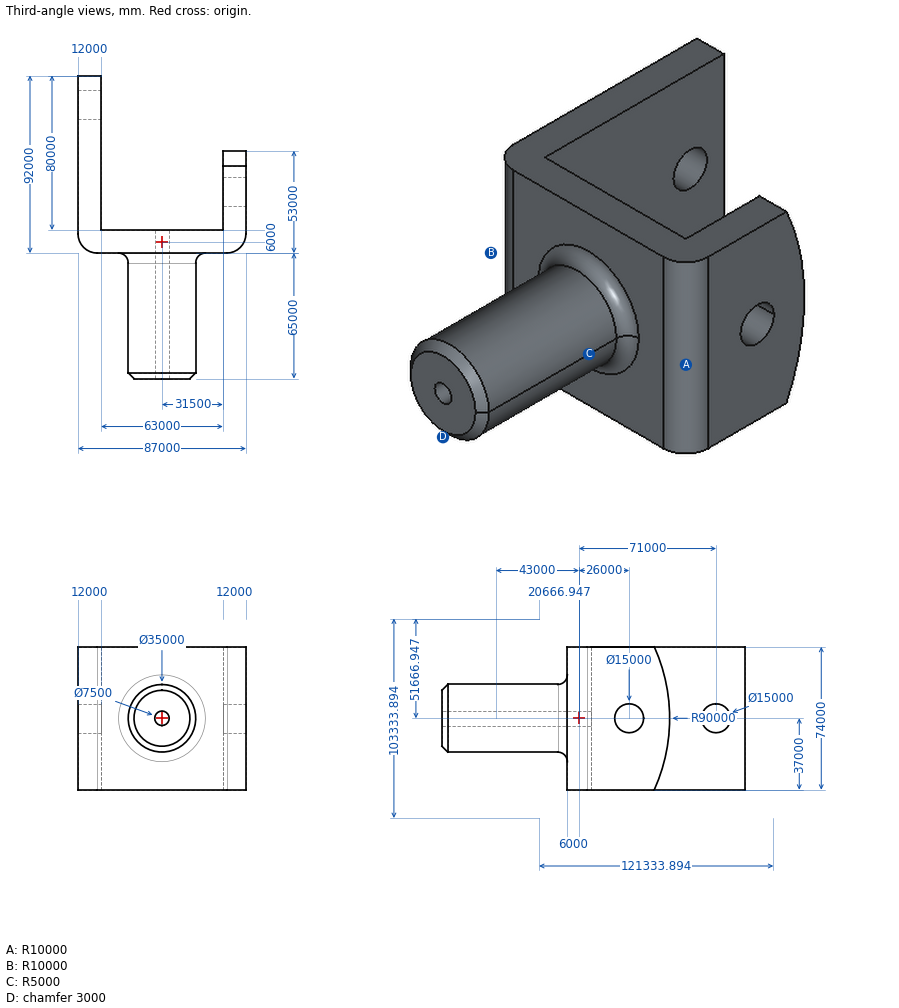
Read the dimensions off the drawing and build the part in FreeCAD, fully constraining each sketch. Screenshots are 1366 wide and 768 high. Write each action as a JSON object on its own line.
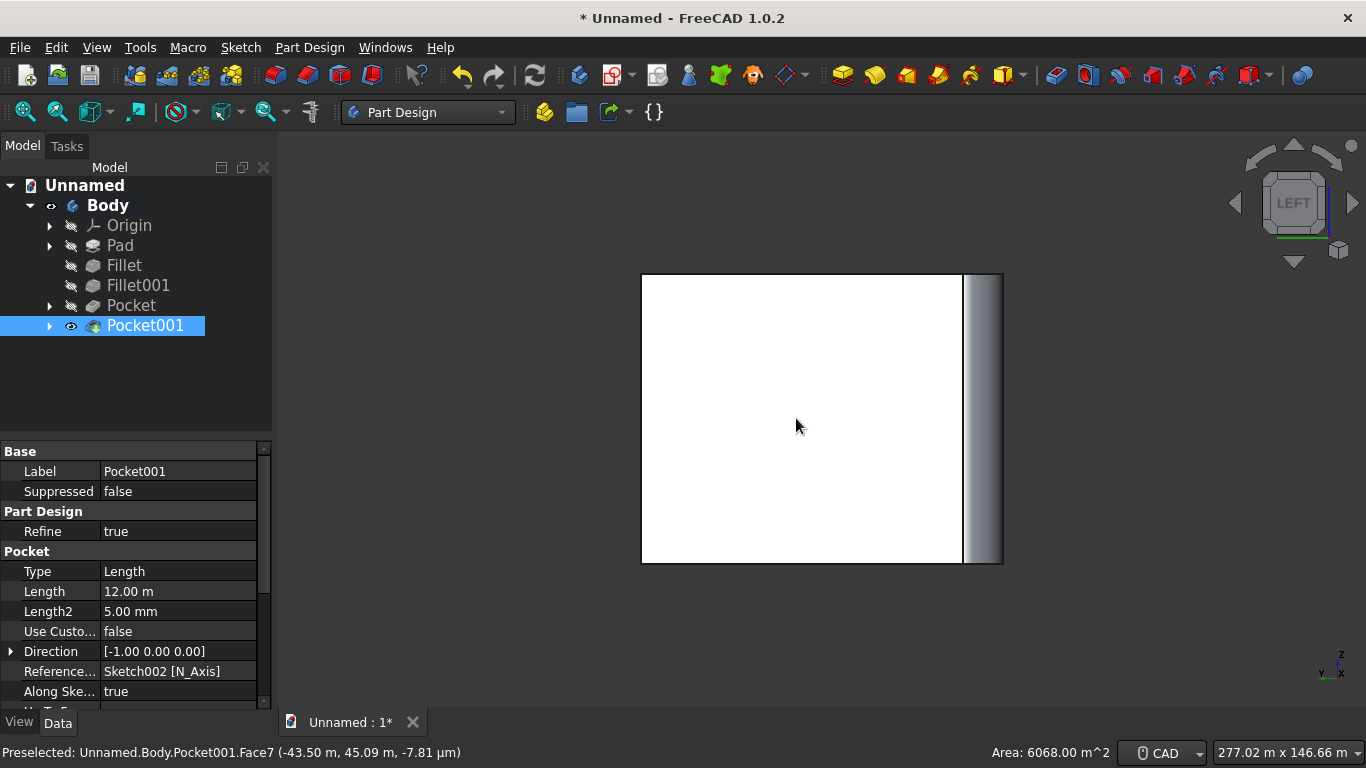
{"action": "left_click", "coordinate": [612, 76]}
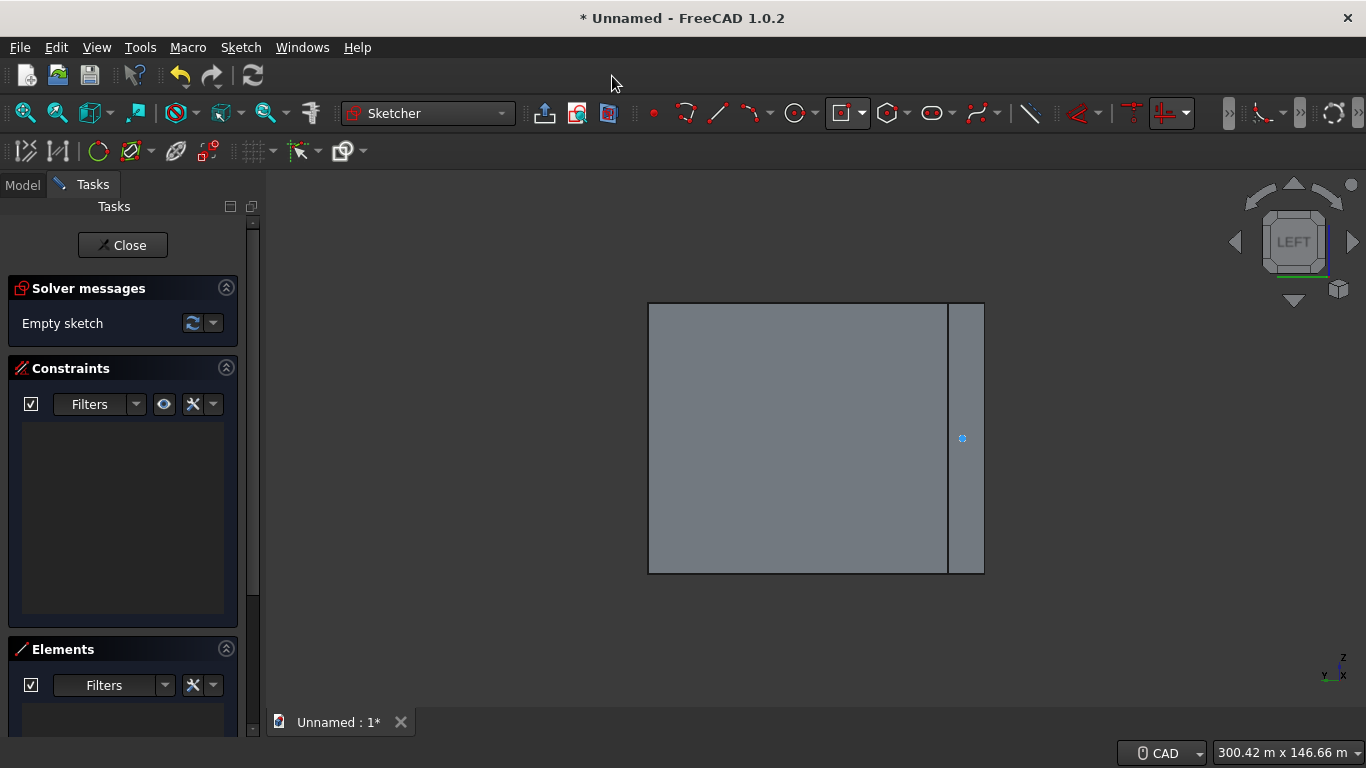
{"action": "scroll", "coordinate": [694, 438], "scroll_direction": "up", "scroll_amount": 9}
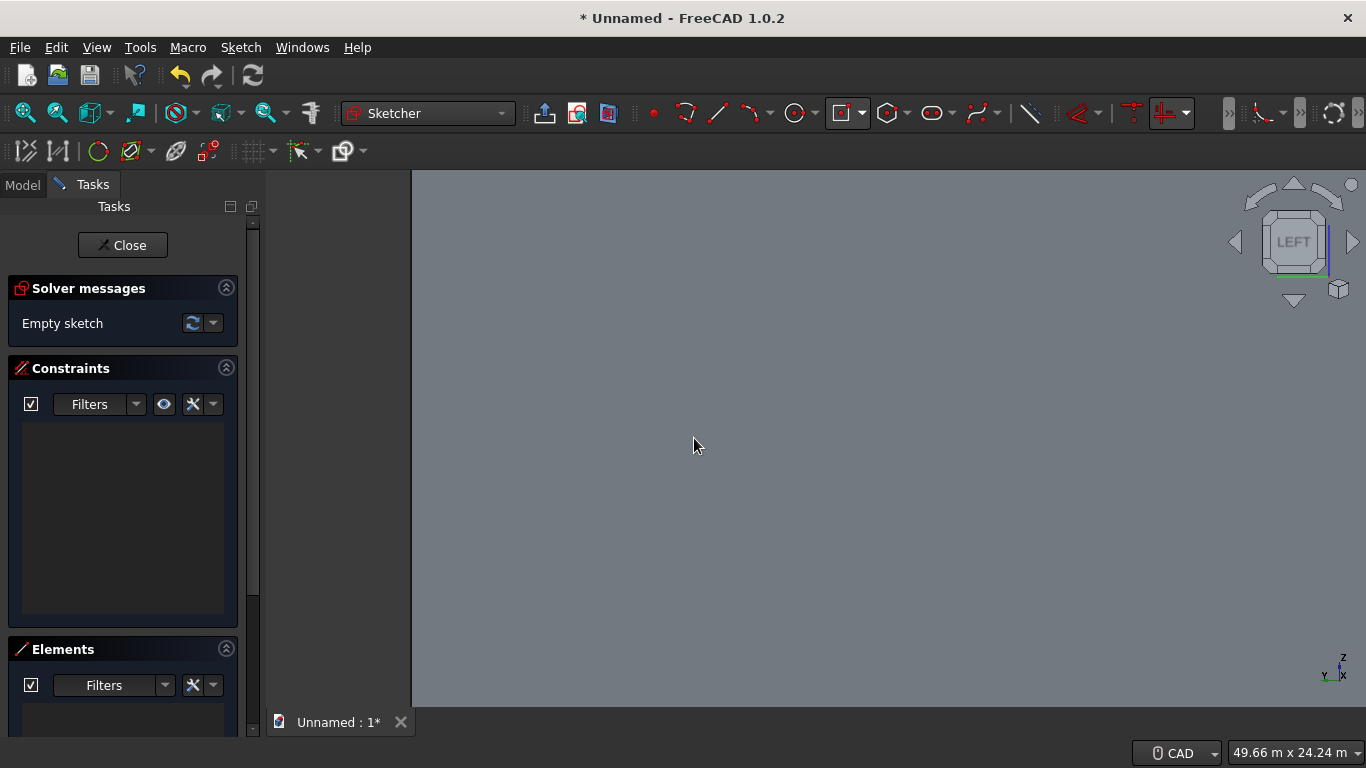
{"action": "key", "text": "g c"}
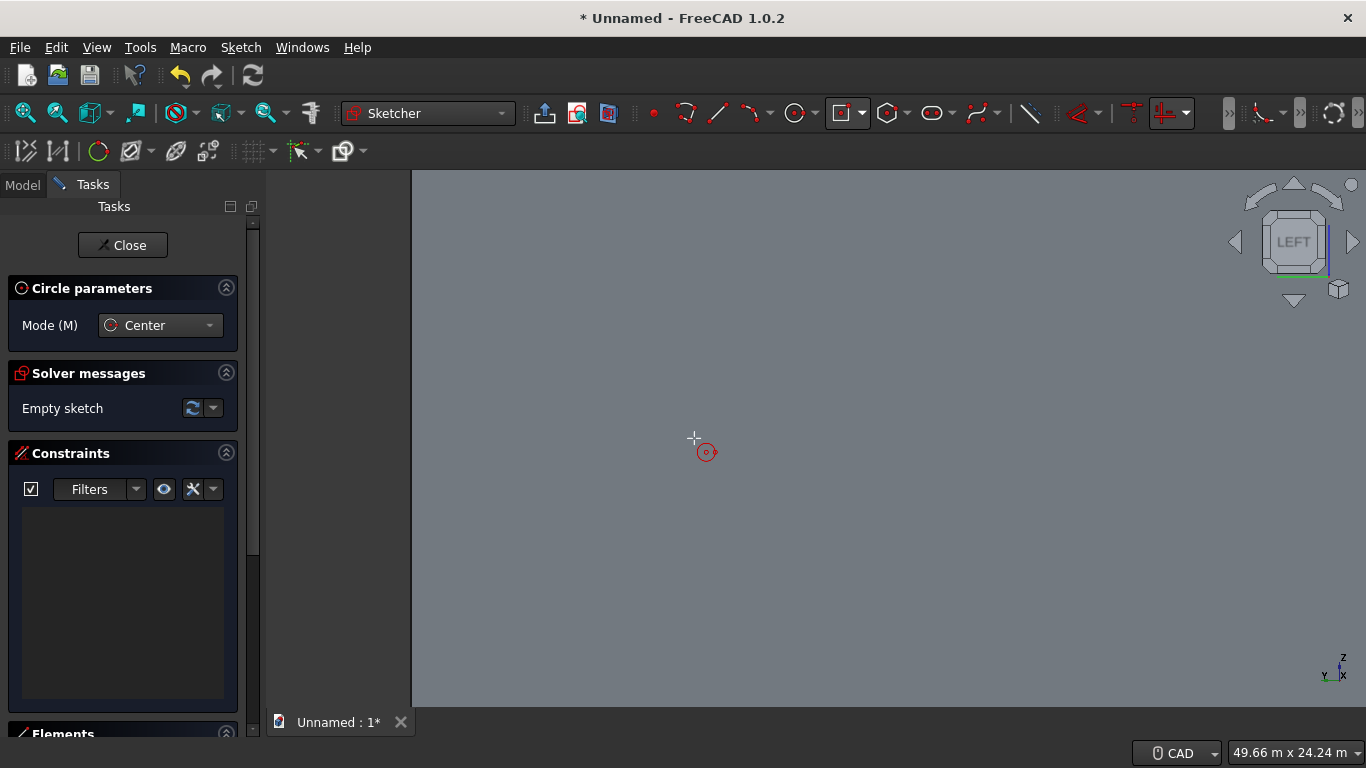
{"action": "left_click", "coordinate": [743, 438]}
{"action": "left_click", "coordinate": [861, 321]}
{"action": "key", "text": "Escape"}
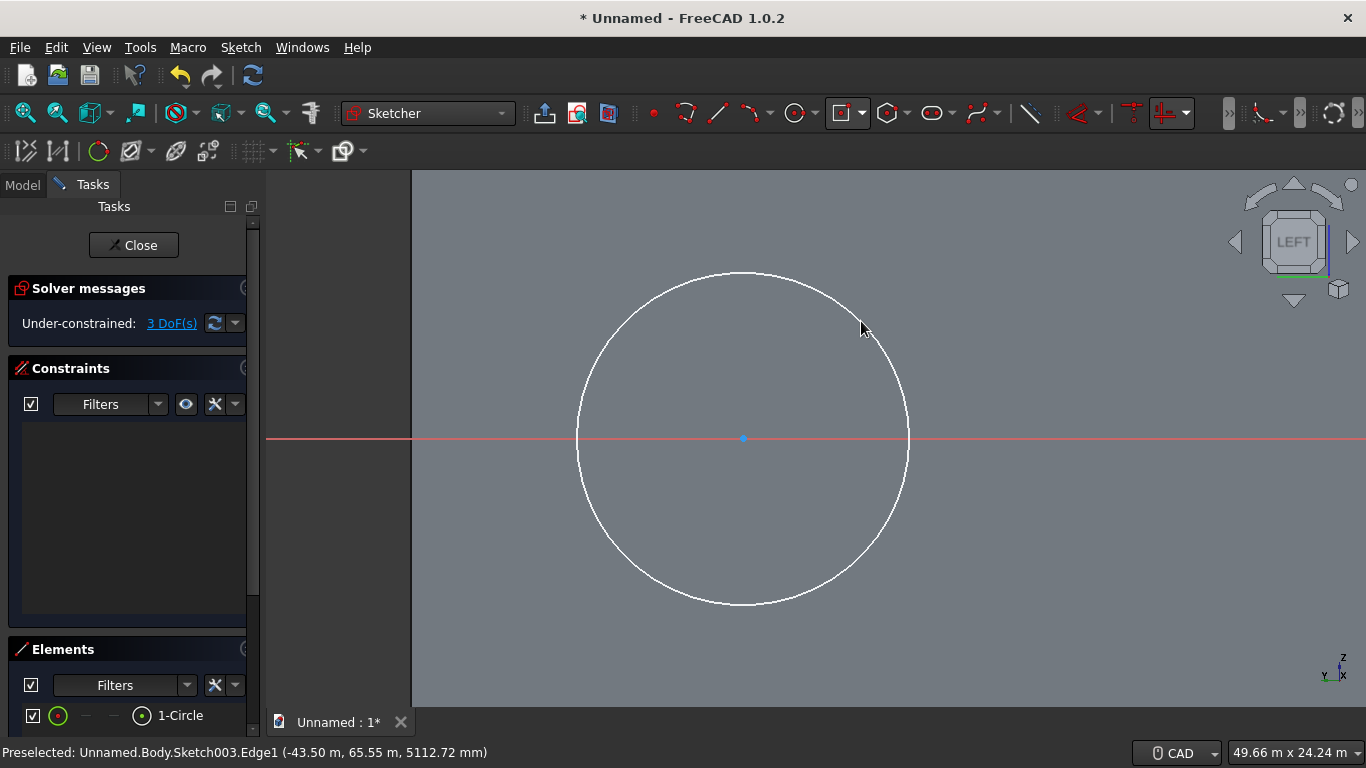
{"action": "left_click", "coordinate": [743, 439]}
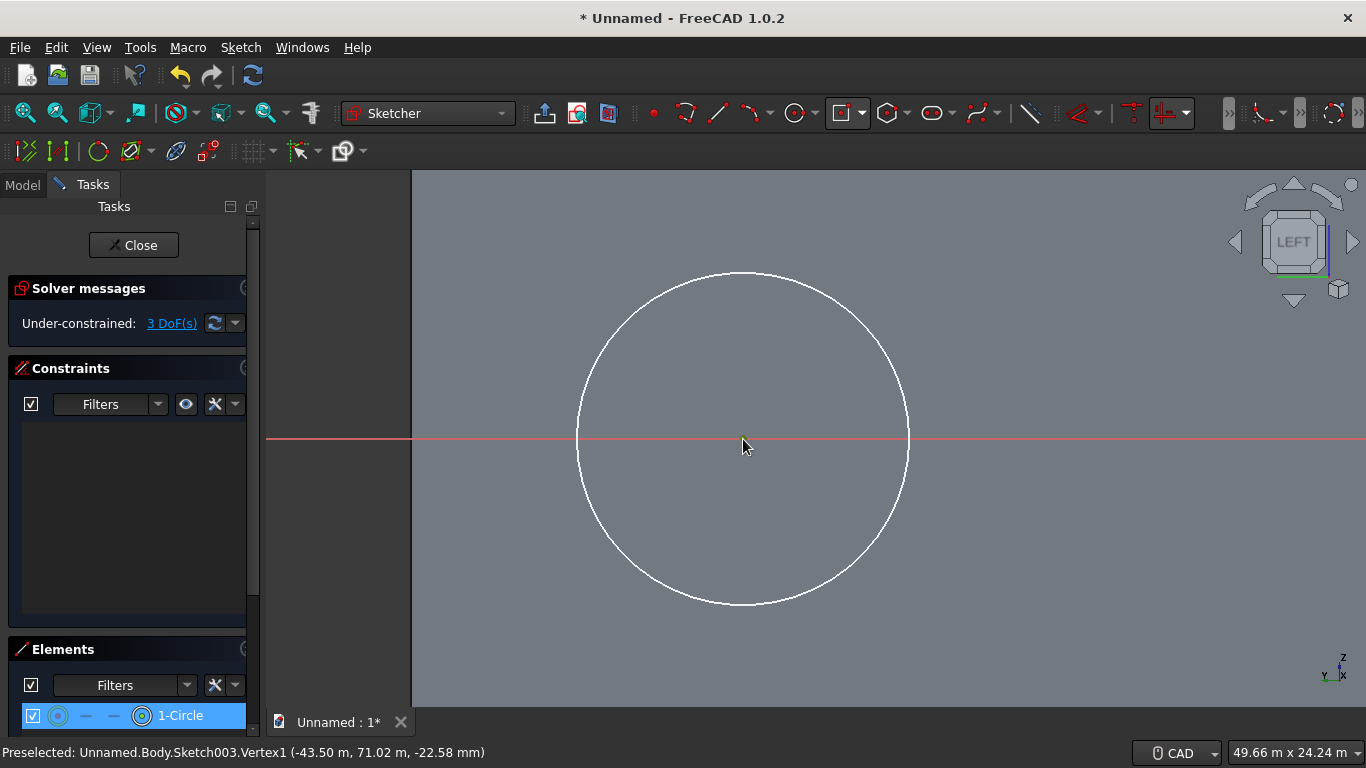
{"action": "left_click", "coordinate": [359, 438]}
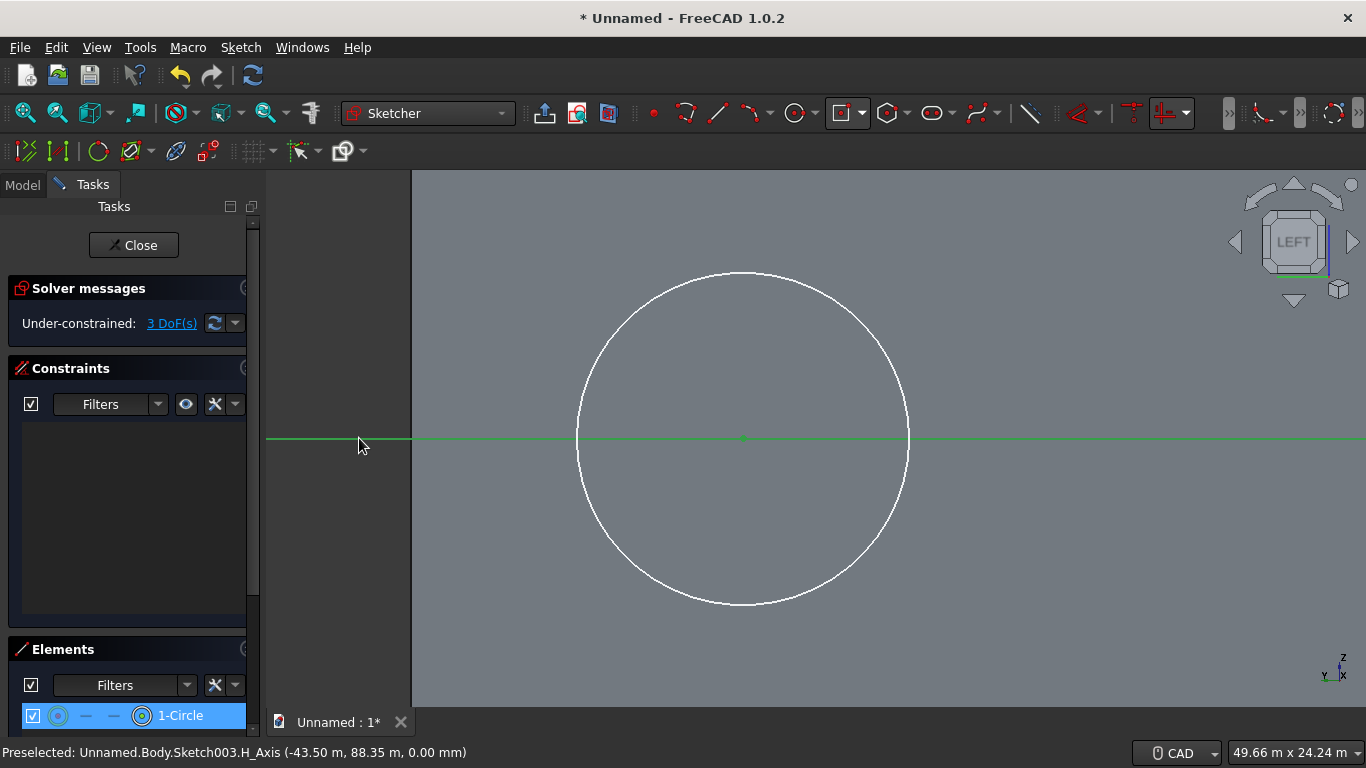
{"action": "left_click", "coordinate": [1132, 114]}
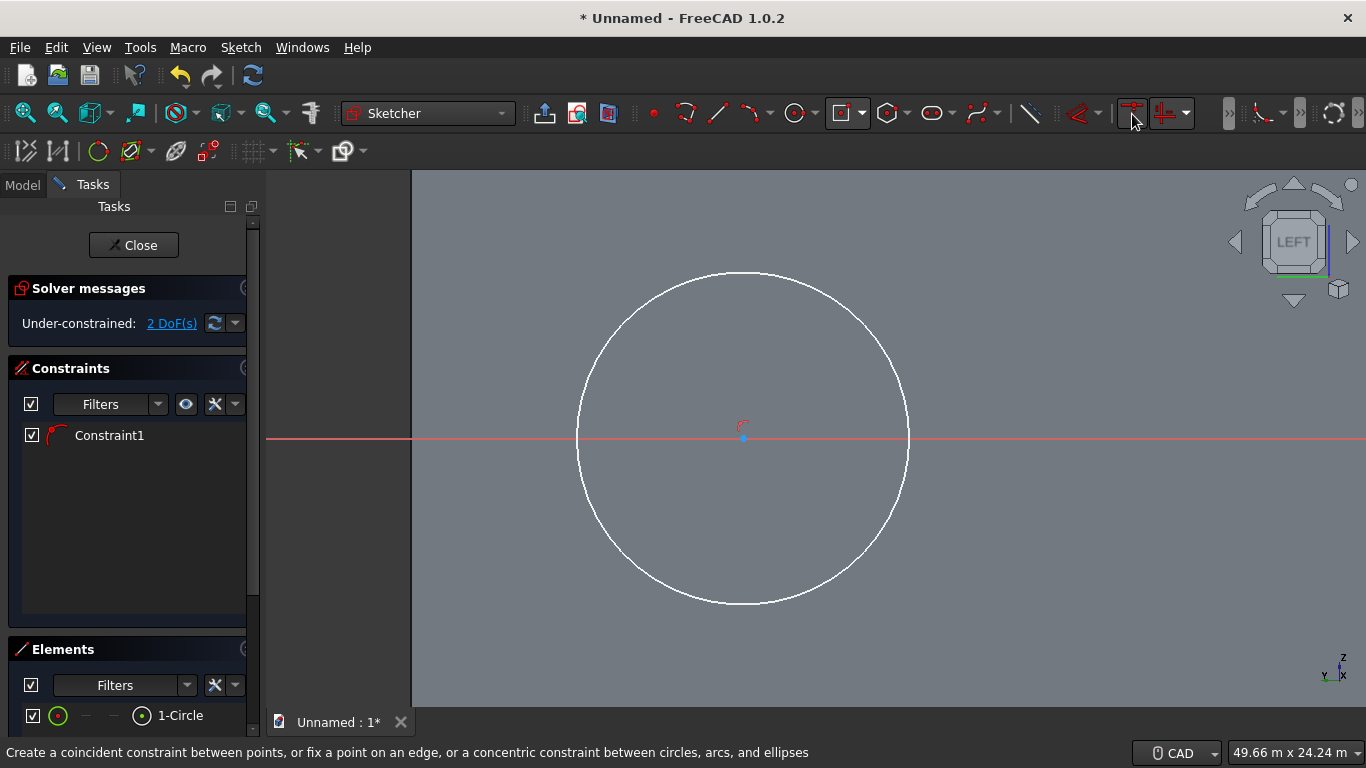
{"action": "left_click", "coordinate": [1078, 114]}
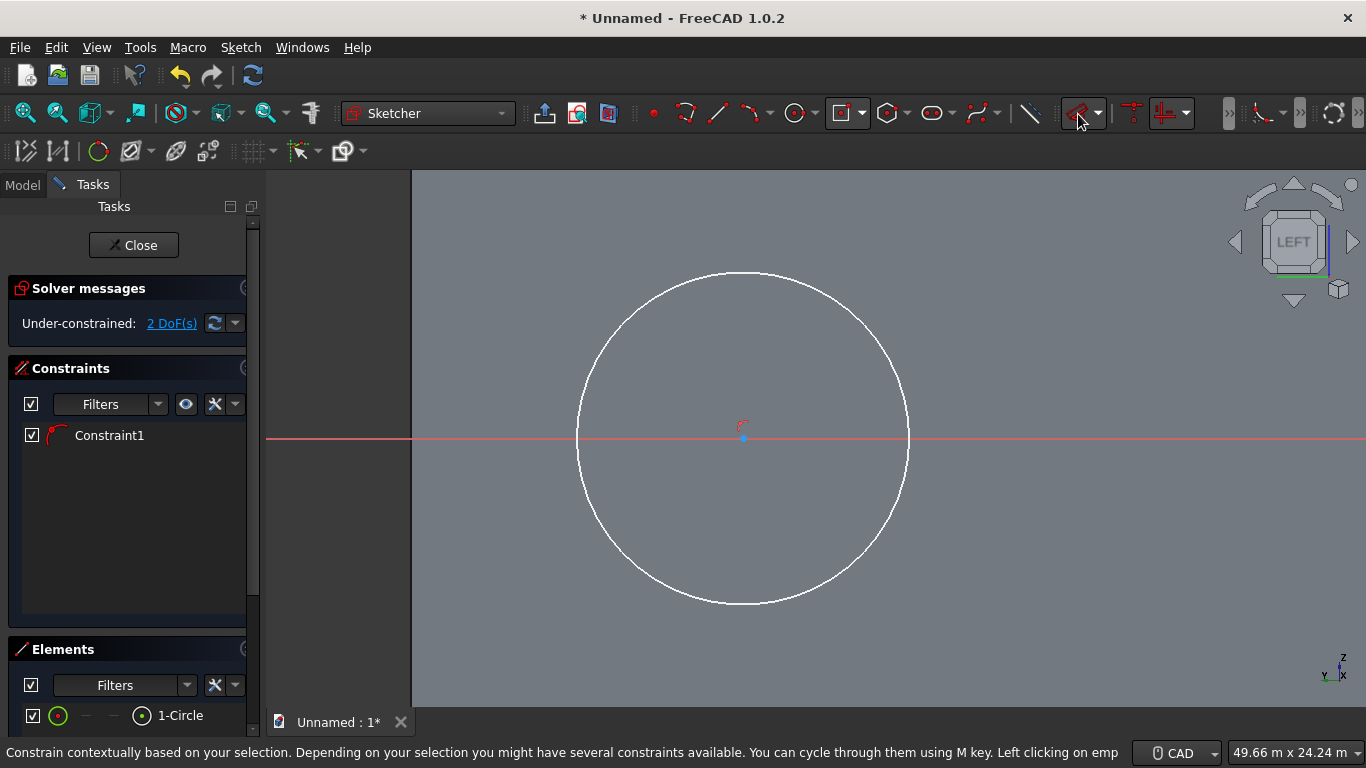
{"action": "left_click", "coordinate": [860, 321]}
{"action": "left_click", "coordinate": [883, 298]}